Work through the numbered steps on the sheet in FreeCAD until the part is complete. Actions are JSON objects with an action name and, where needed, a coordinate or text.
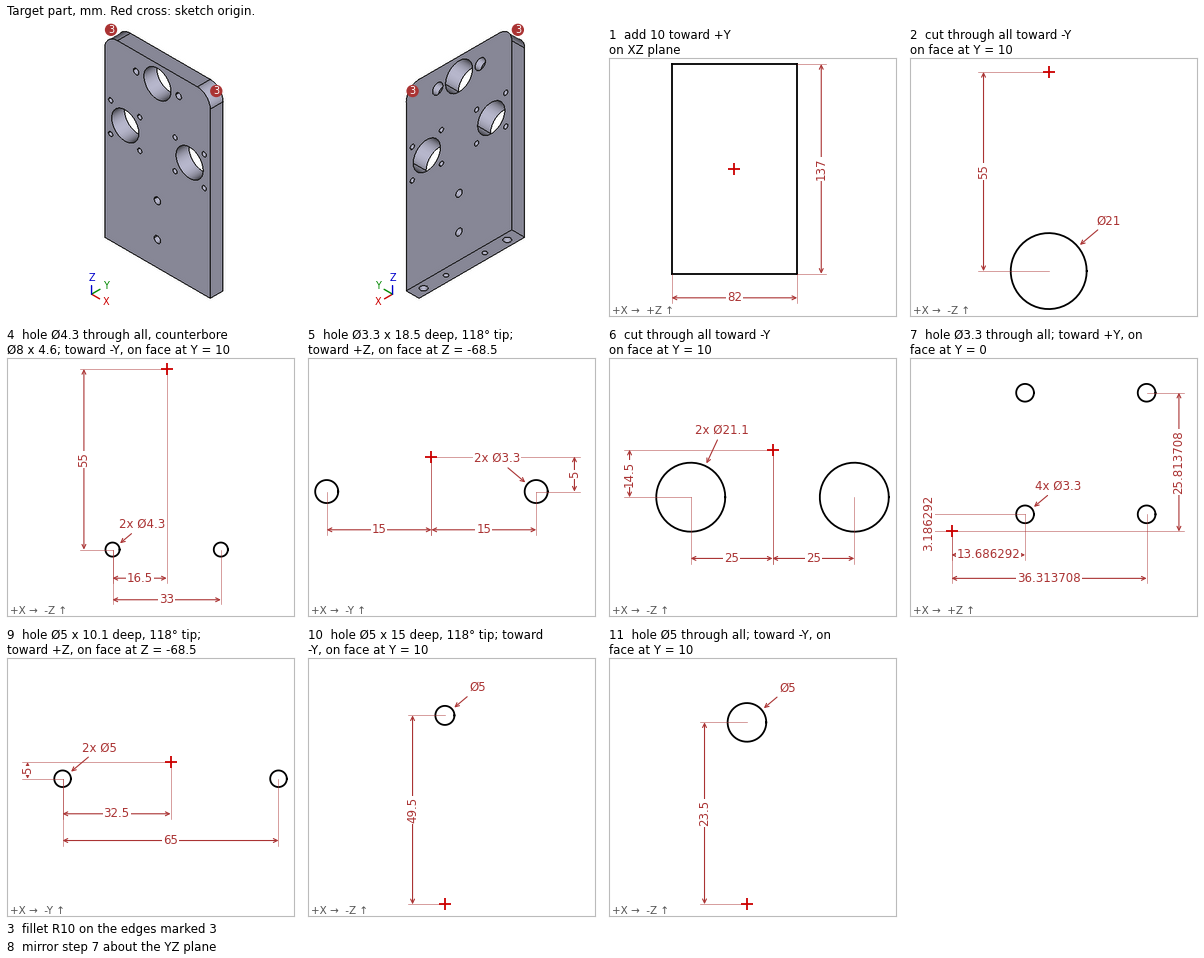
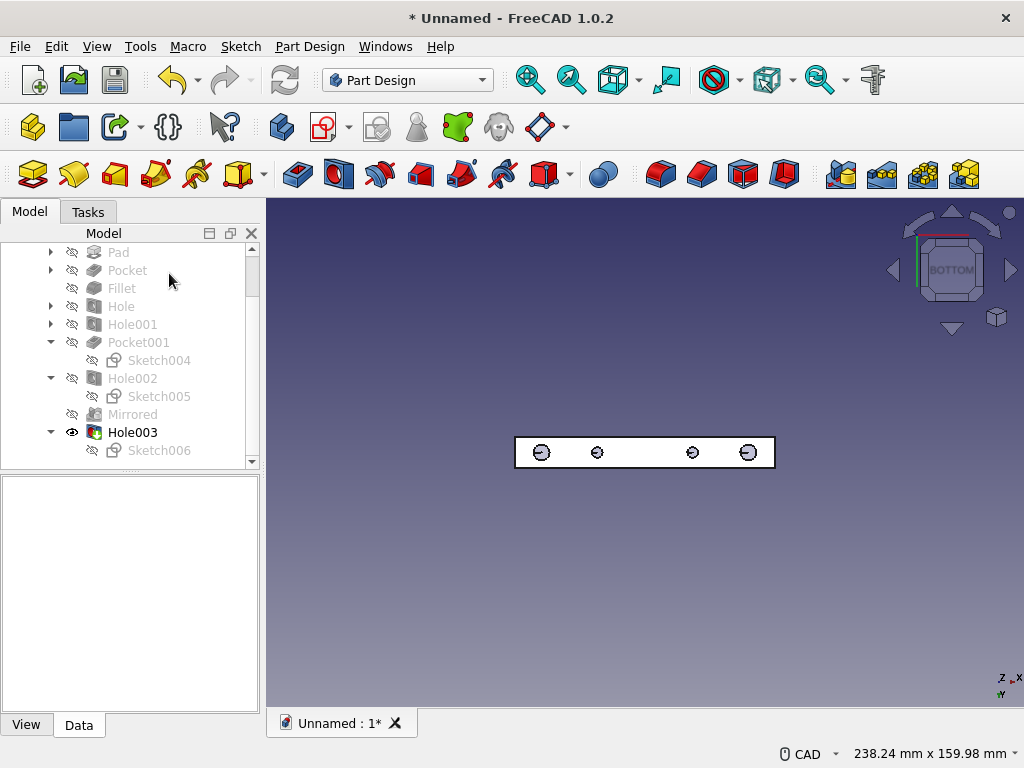
{"action": "left_click", "coordinate": [531, 80]}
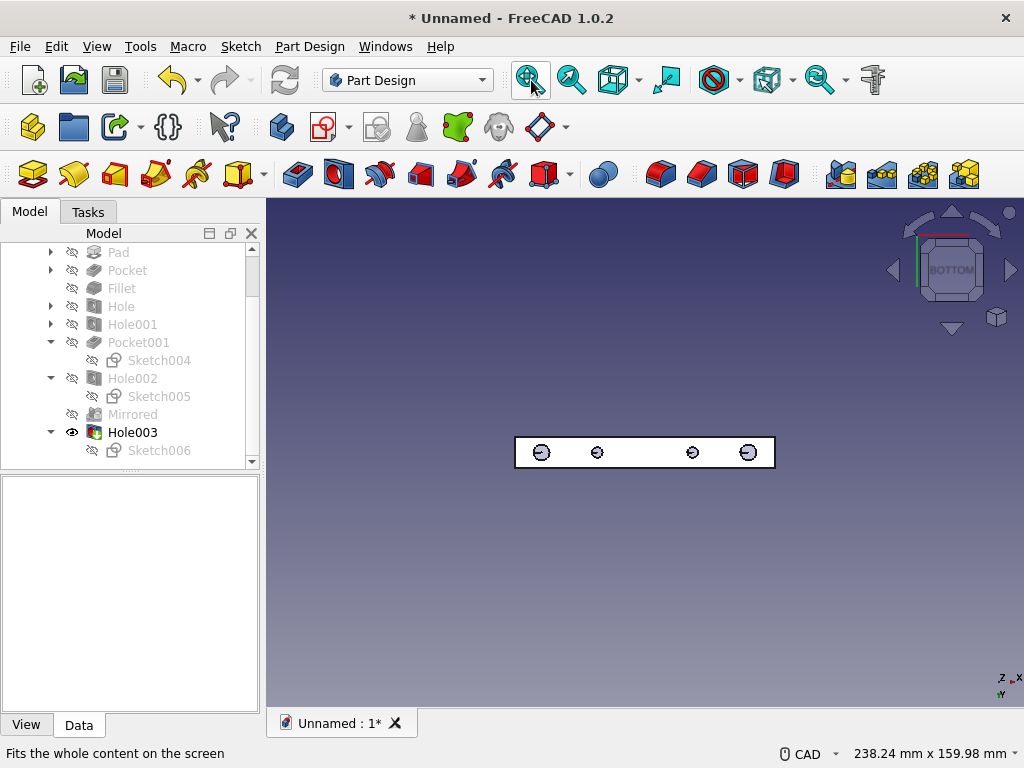
{"action": "key", "text": "4"}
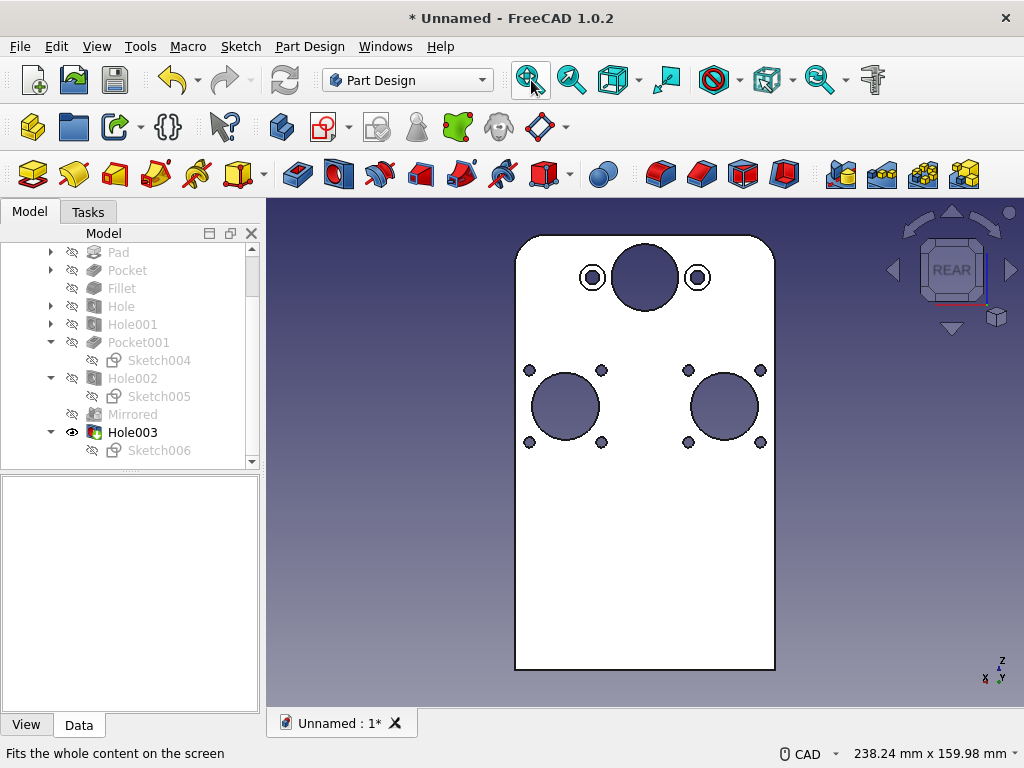
{"action": "left_click", "coordinate": [645, 576]}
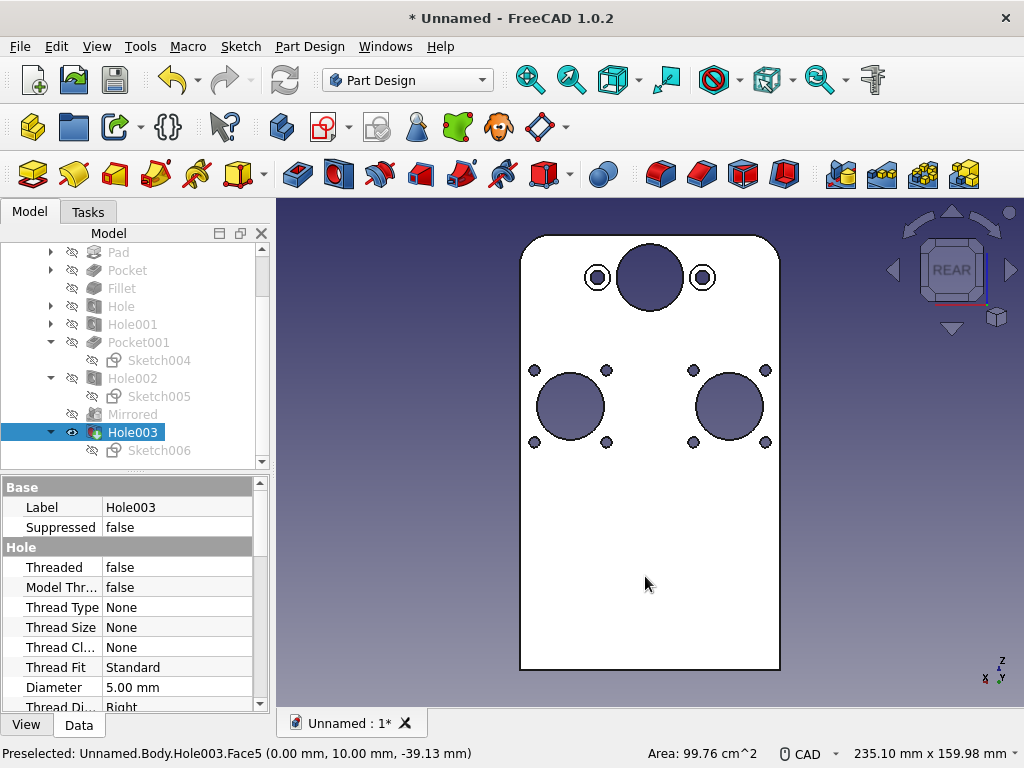
{"action": "left_click", "coordinate": [322, 128]}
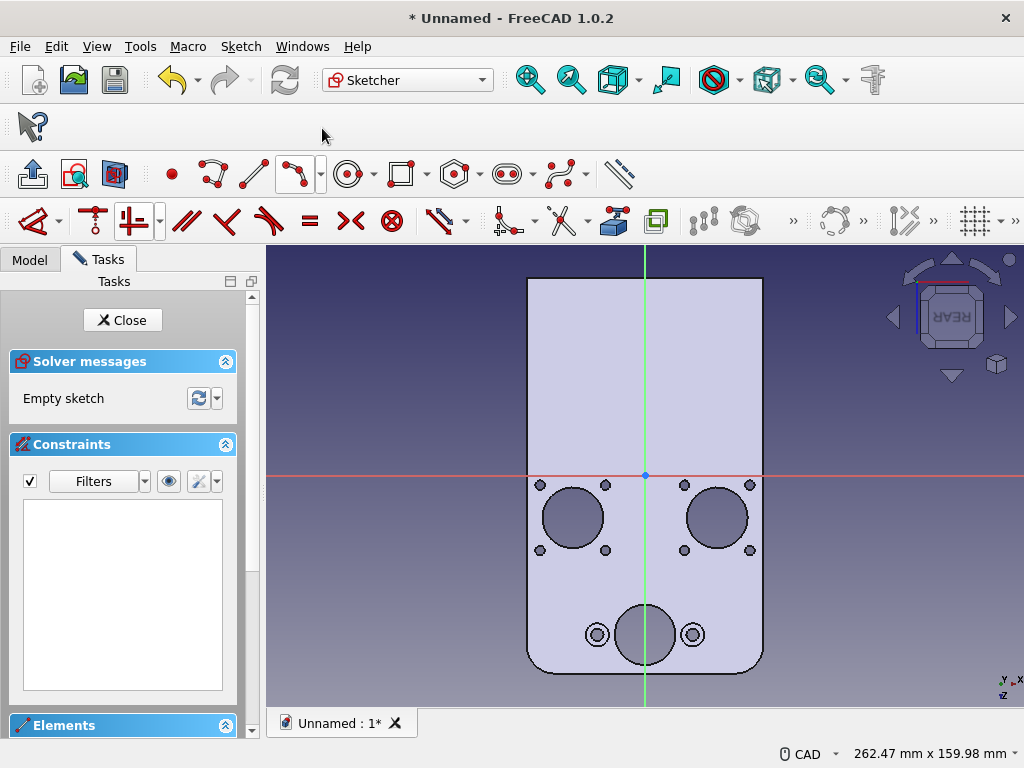
{"action": "scroll", "coordinate": [649, 326], "scroll_direction": "up", "scroll_amount": 15}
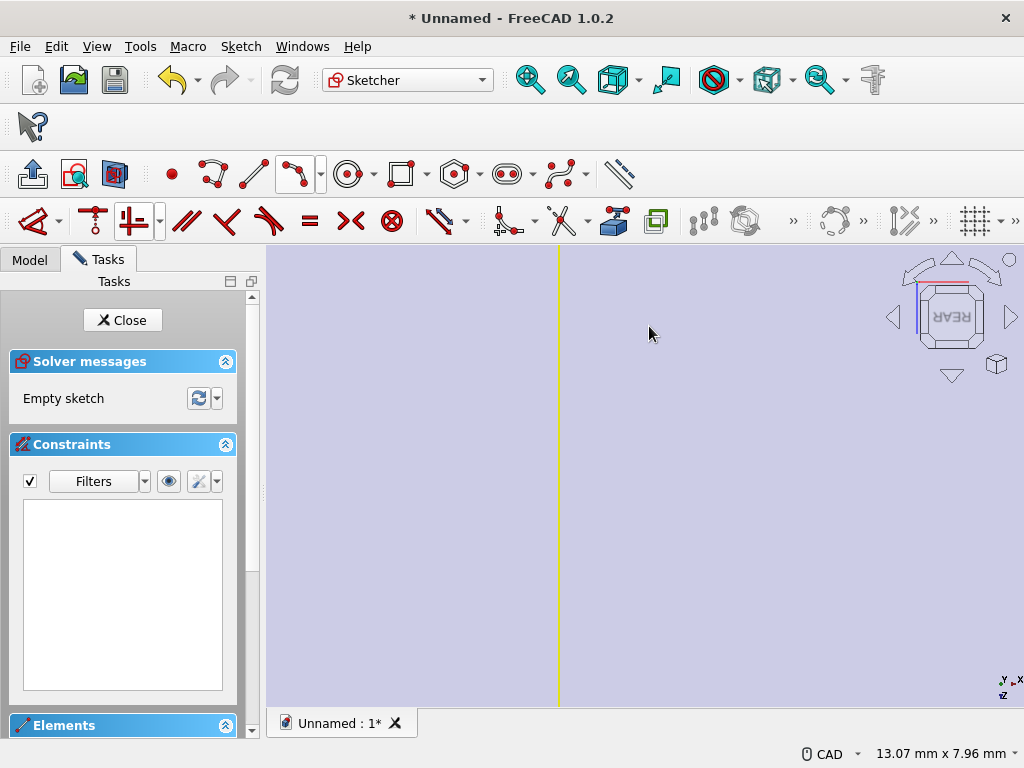
{"action": "key", "text": "g c"}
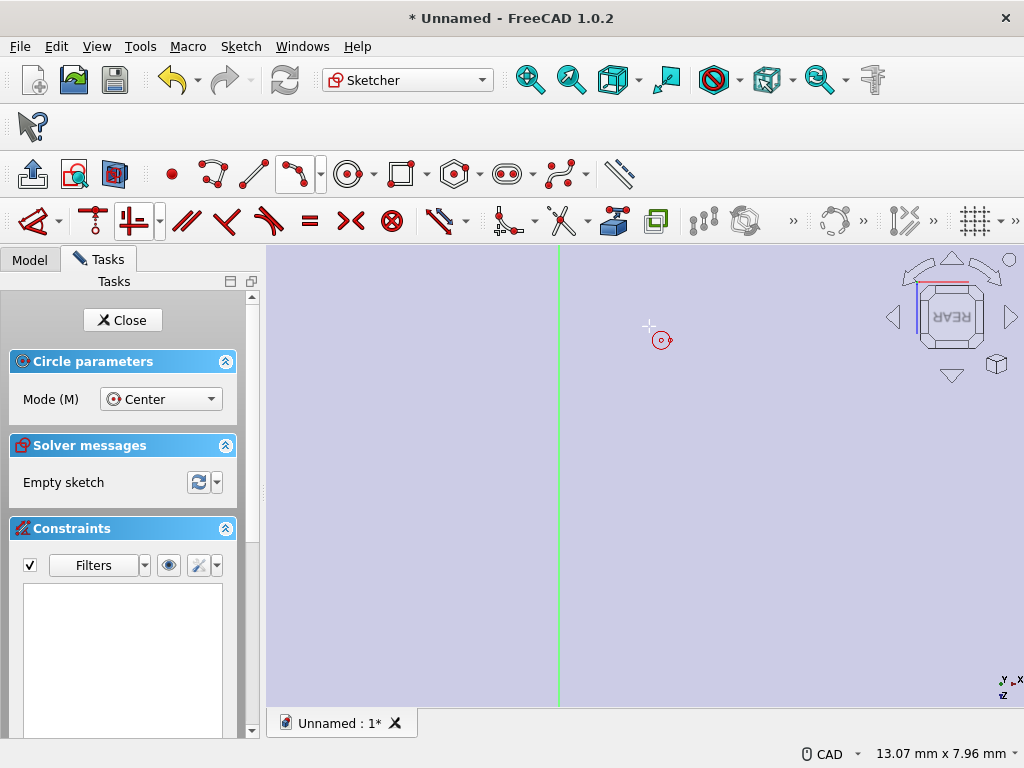
{"action": "left_click", "coordinate": [559, 464]}
{"action": "mouse_move", "coordinate": [662, 362]}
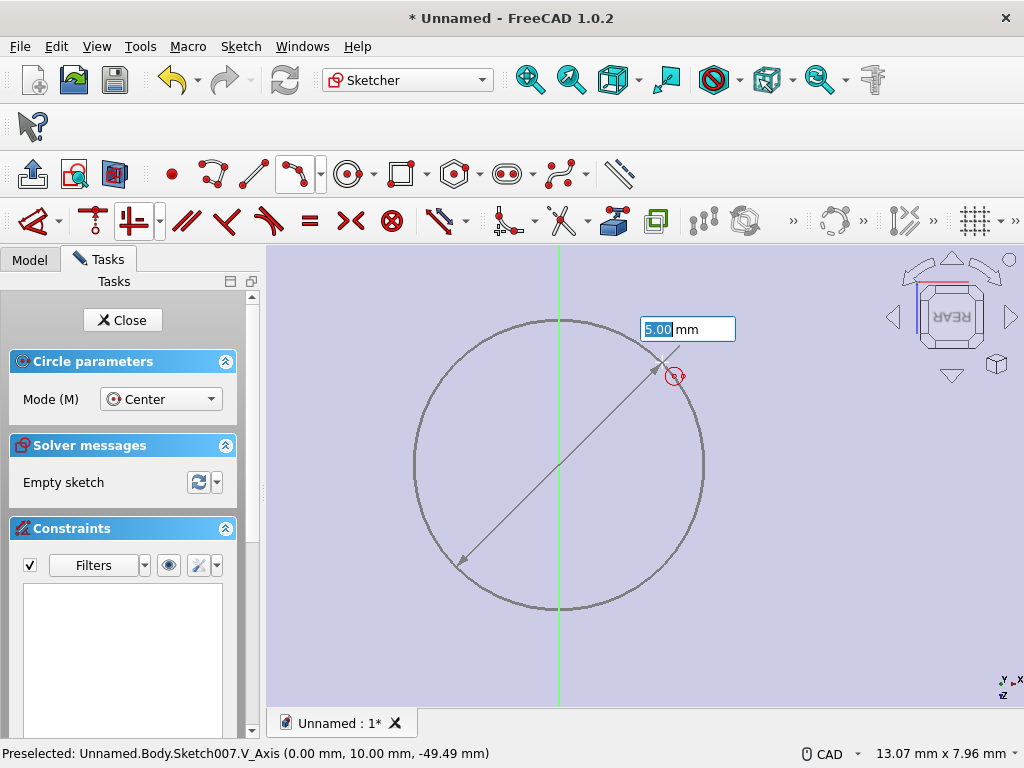
{"action": "type", "text": "5"}
{"action": "key", "text": "Return"}
{"action": "key", "text": "Escape"}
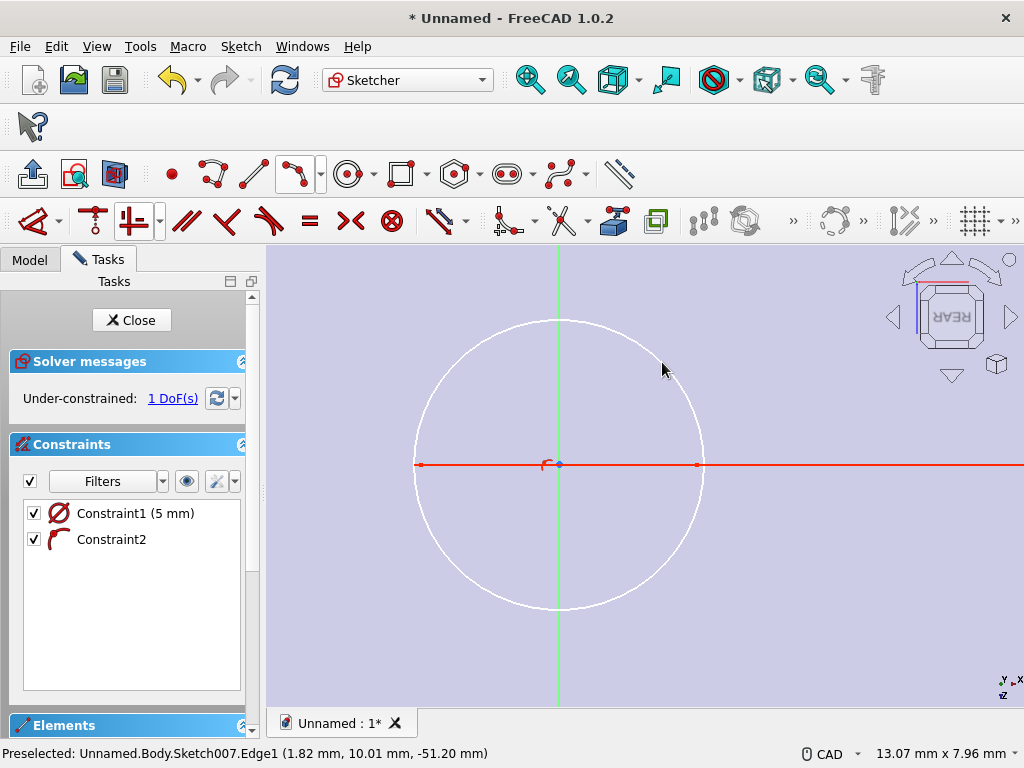
{"action": "key", "text": "d"}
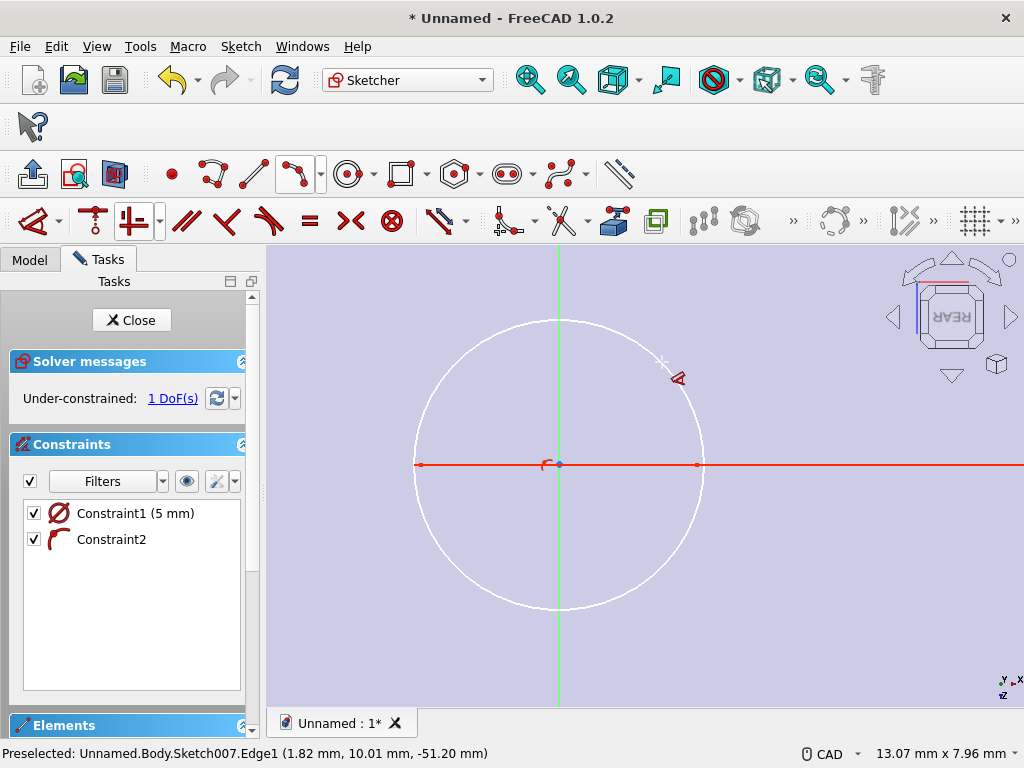
{"action": "left_click", "coordinate": [559, 465]}
{"action": "left_click", "coordinate": [593, 572]}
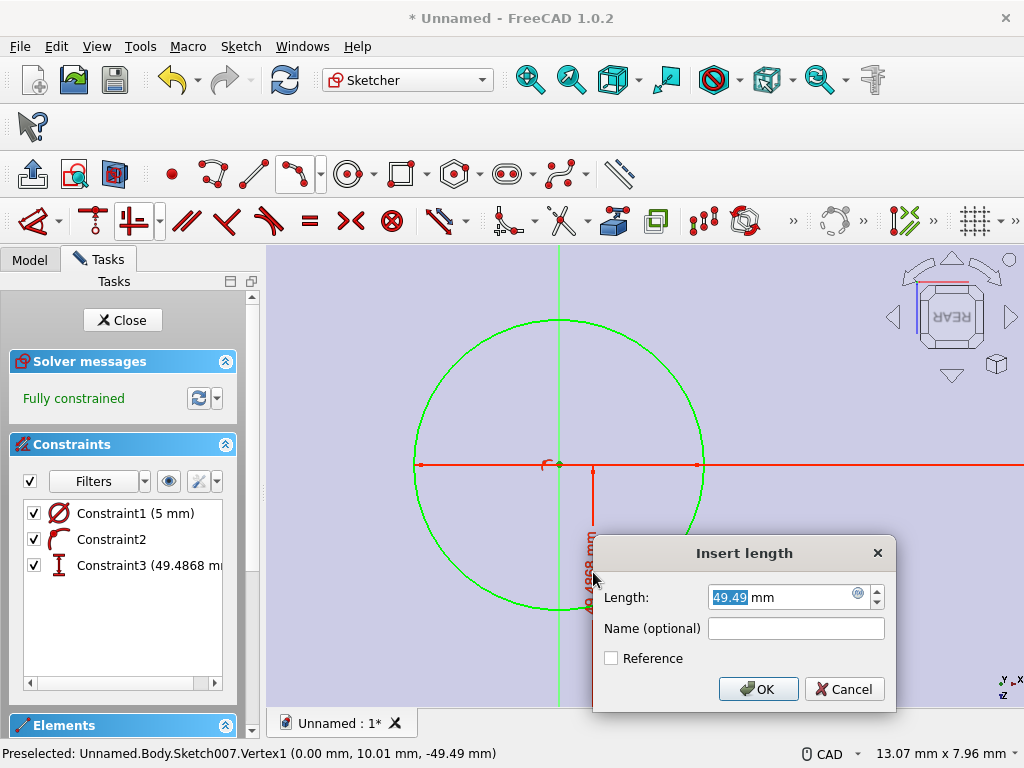
{"action": "type", "text": "49.5"}
{"action": "key", "text": "Return"}
{"action": "key", "text": "Escape"}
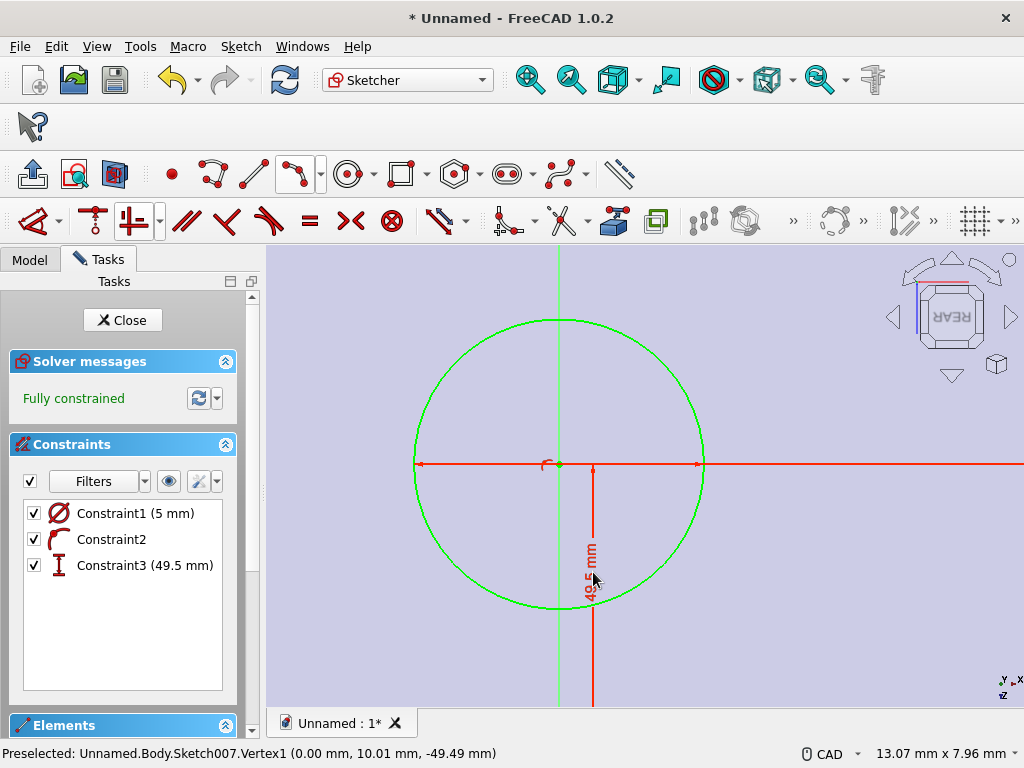
{"action": "left_click", "coordinate": [123, 320]}